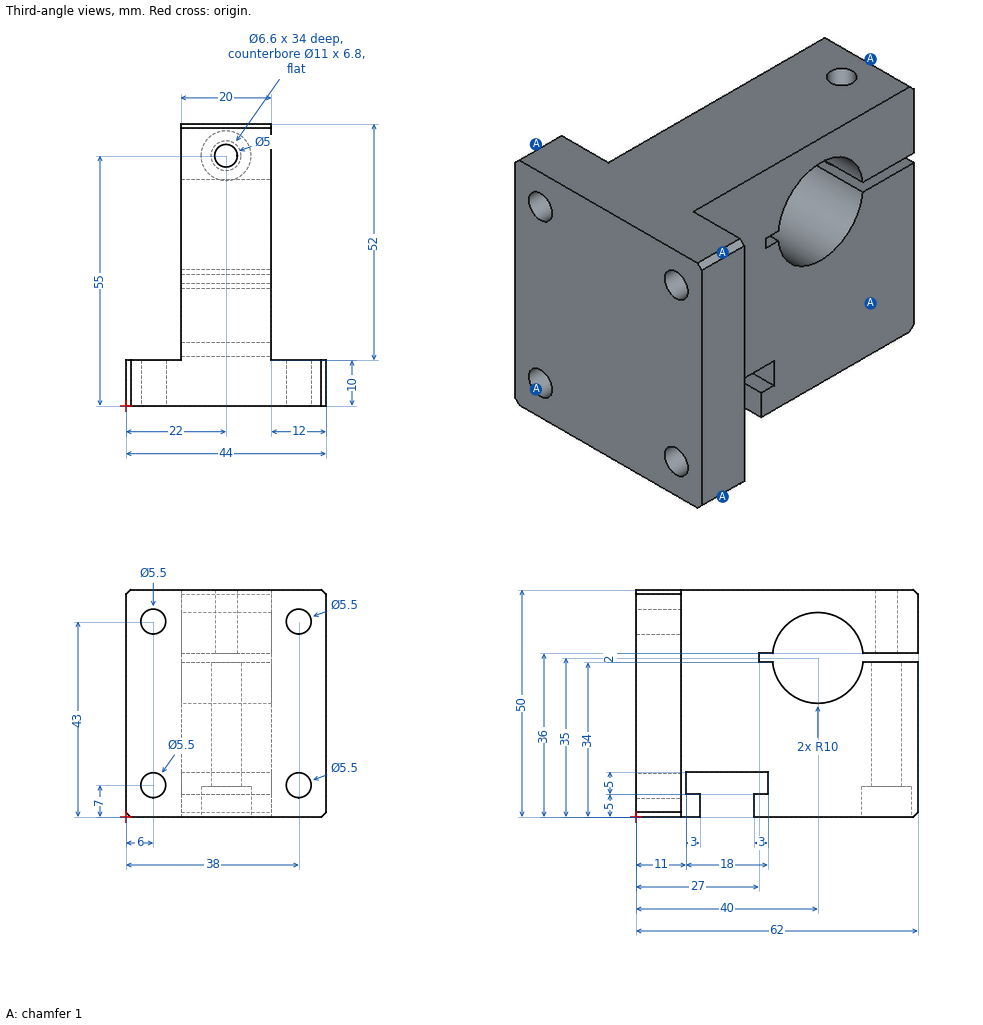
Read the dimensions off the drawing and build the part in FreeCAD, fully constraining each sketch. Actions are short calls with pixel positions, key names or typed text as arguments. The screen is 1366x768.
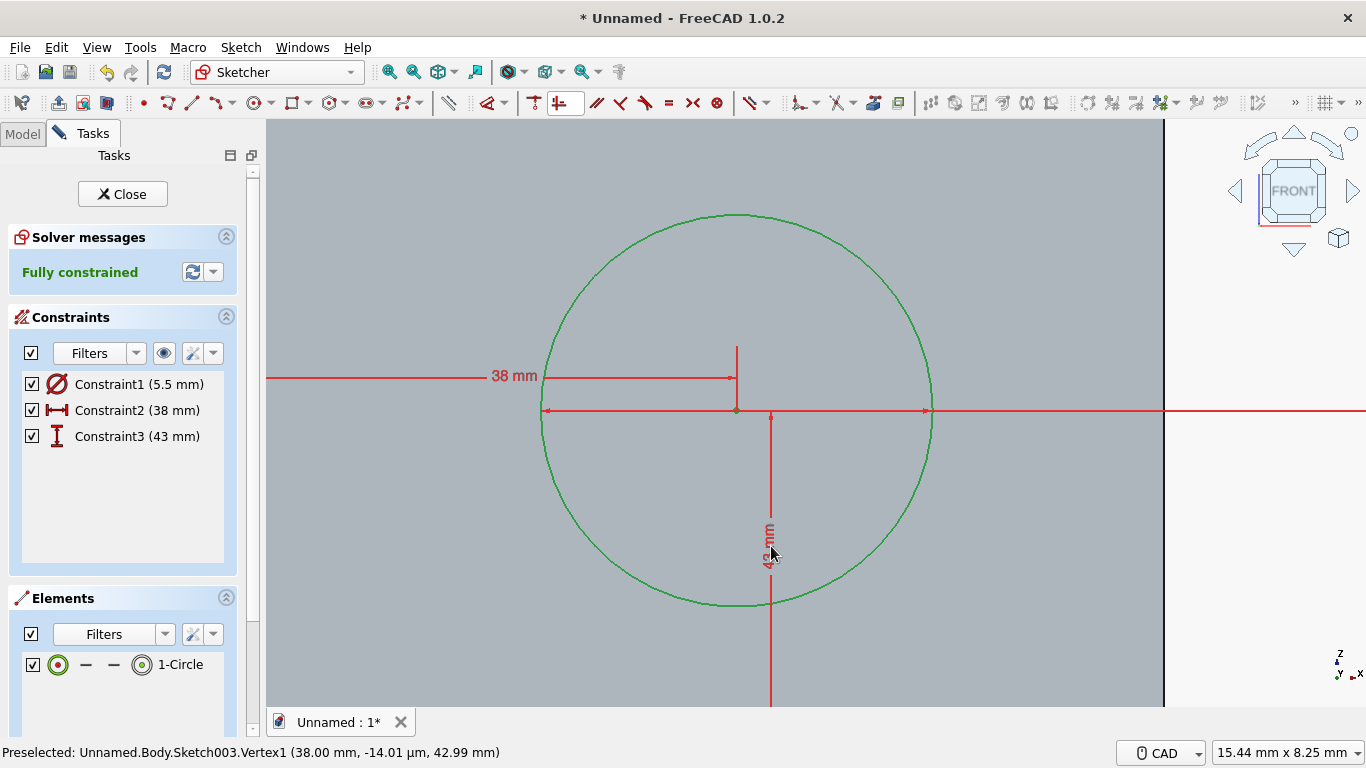
click(123, 194)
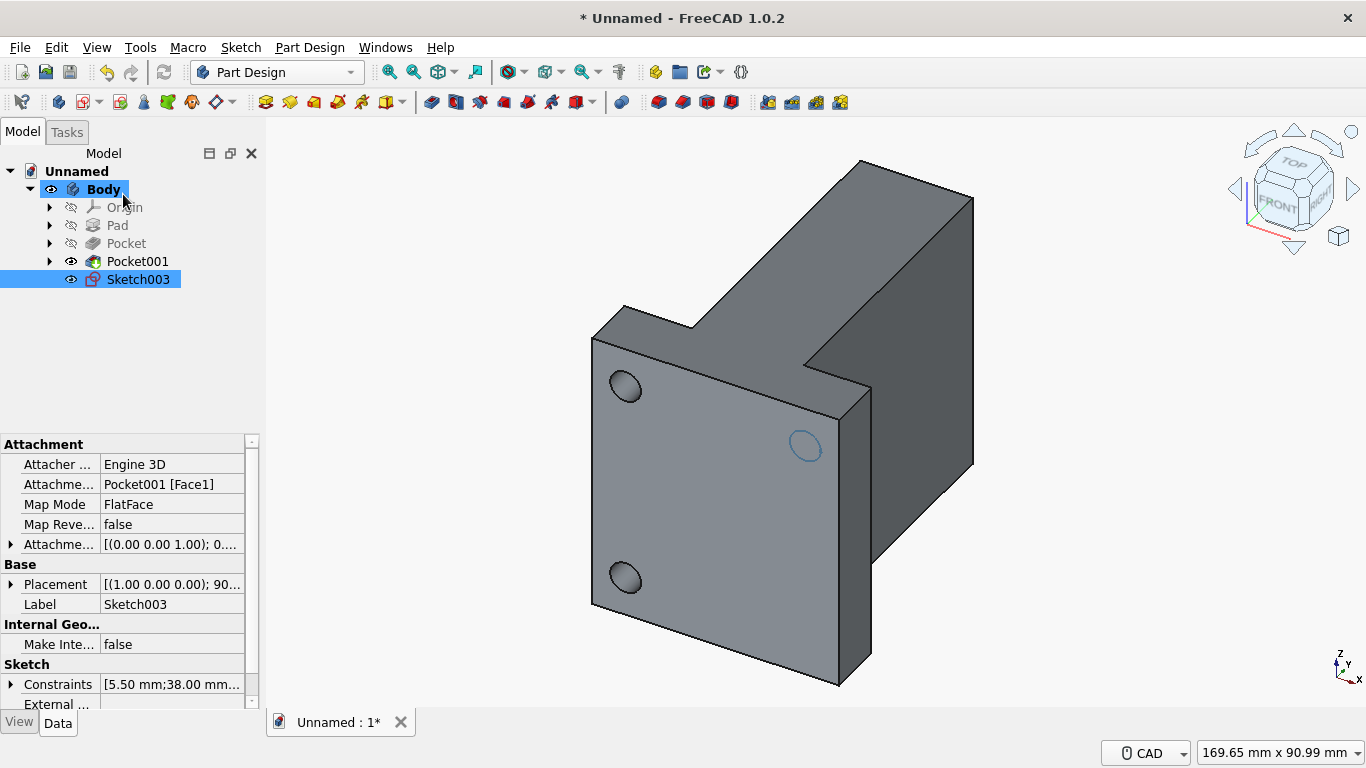
click(432, 102)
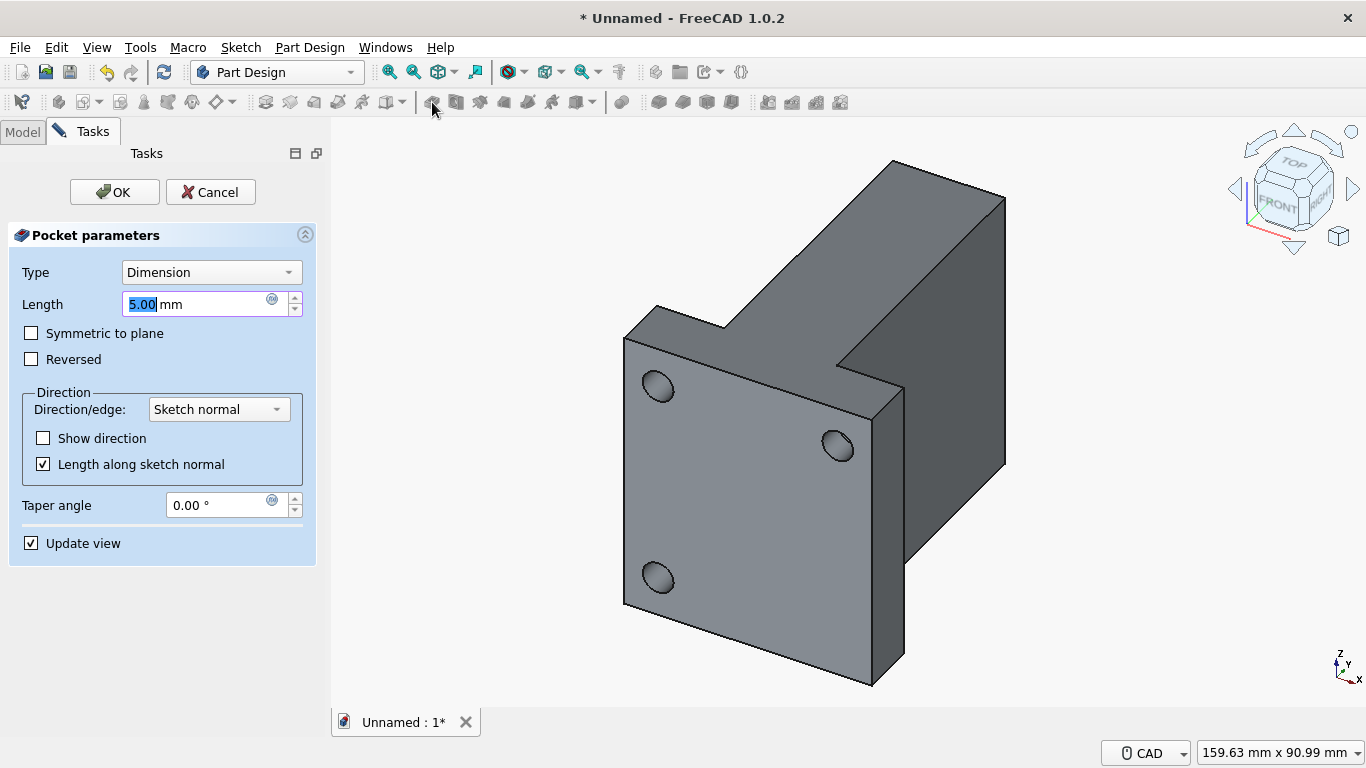
click(212, 272)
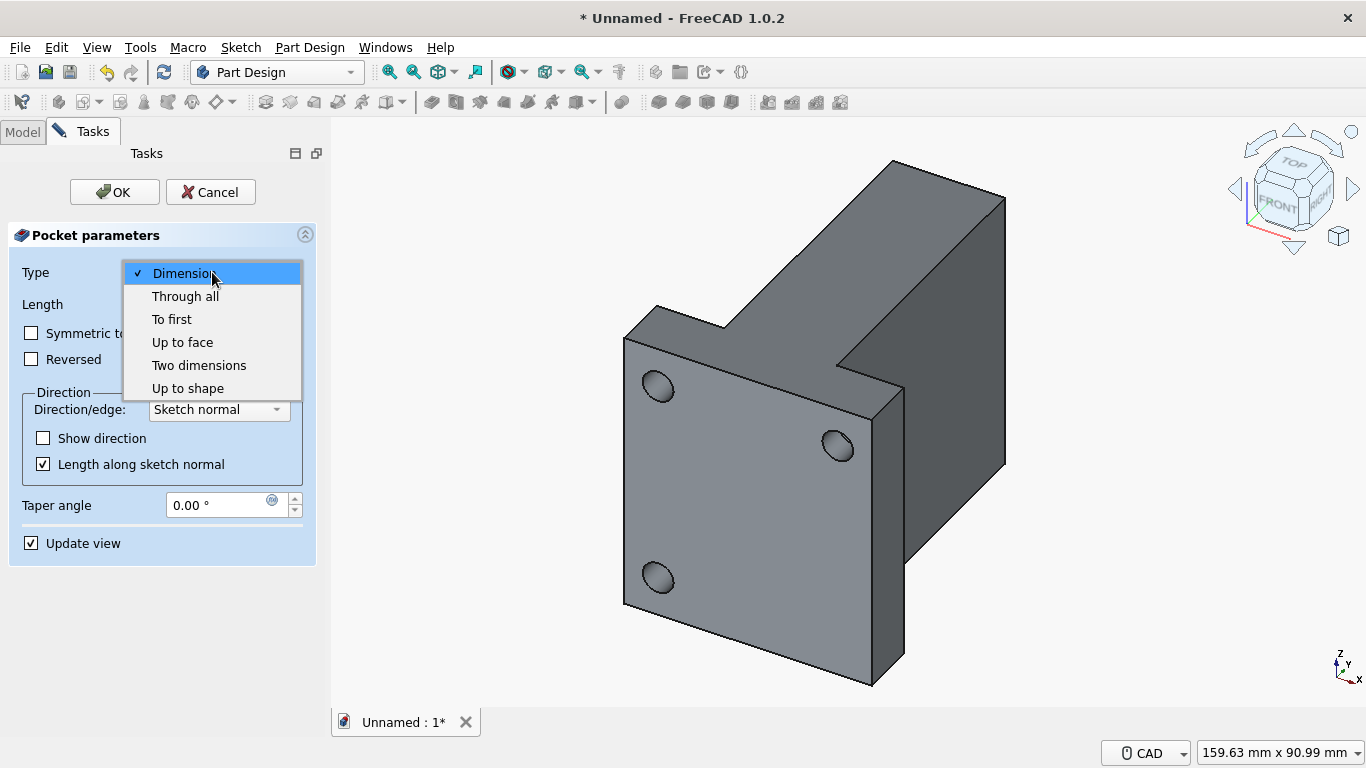
click(212, 320)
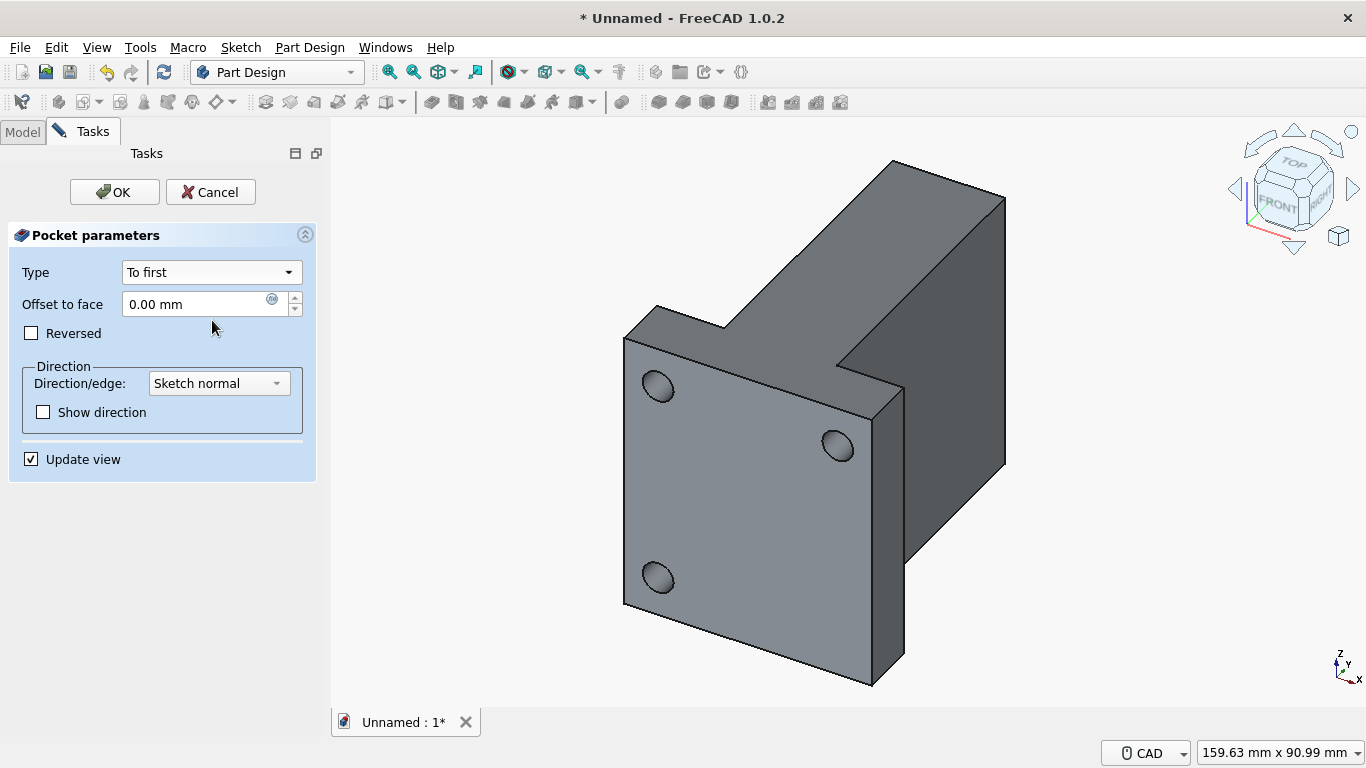
click(115, 192)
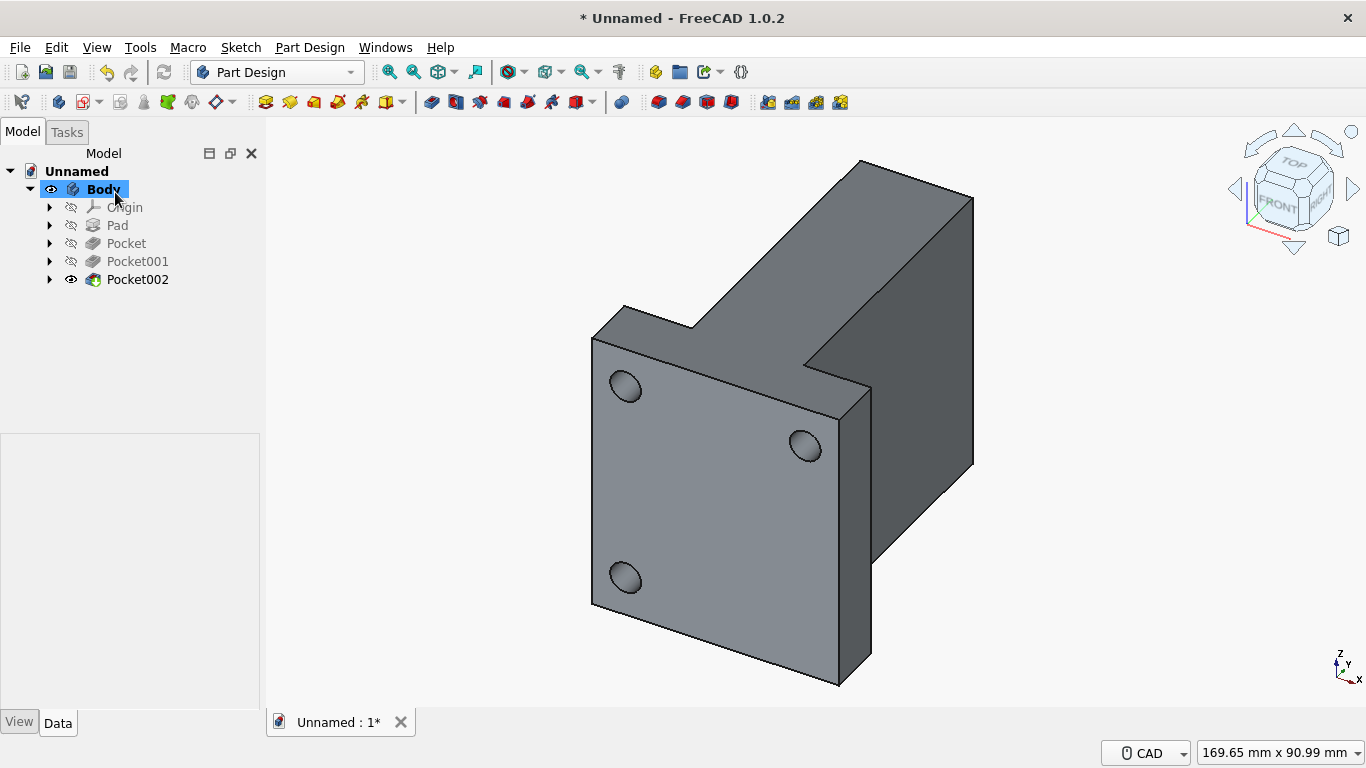
click(84, 102)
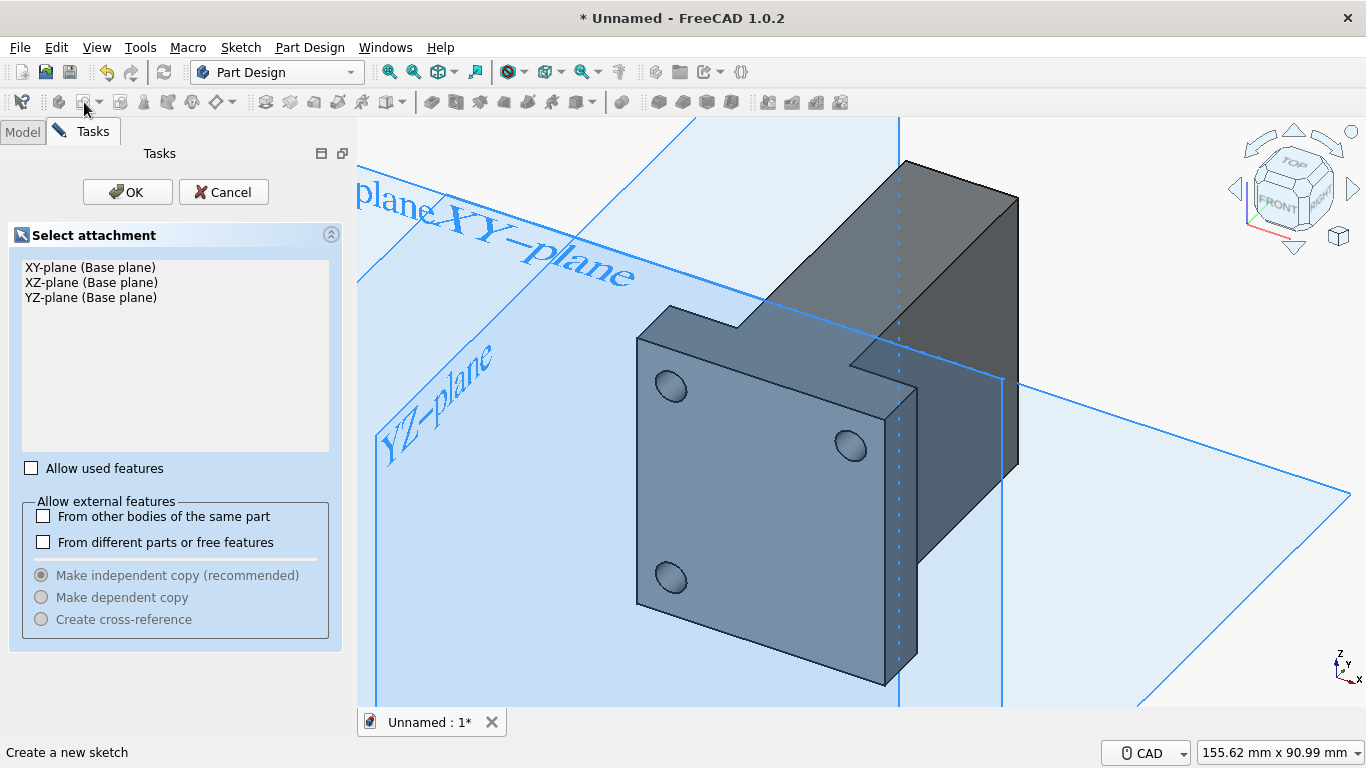
click(82, 282)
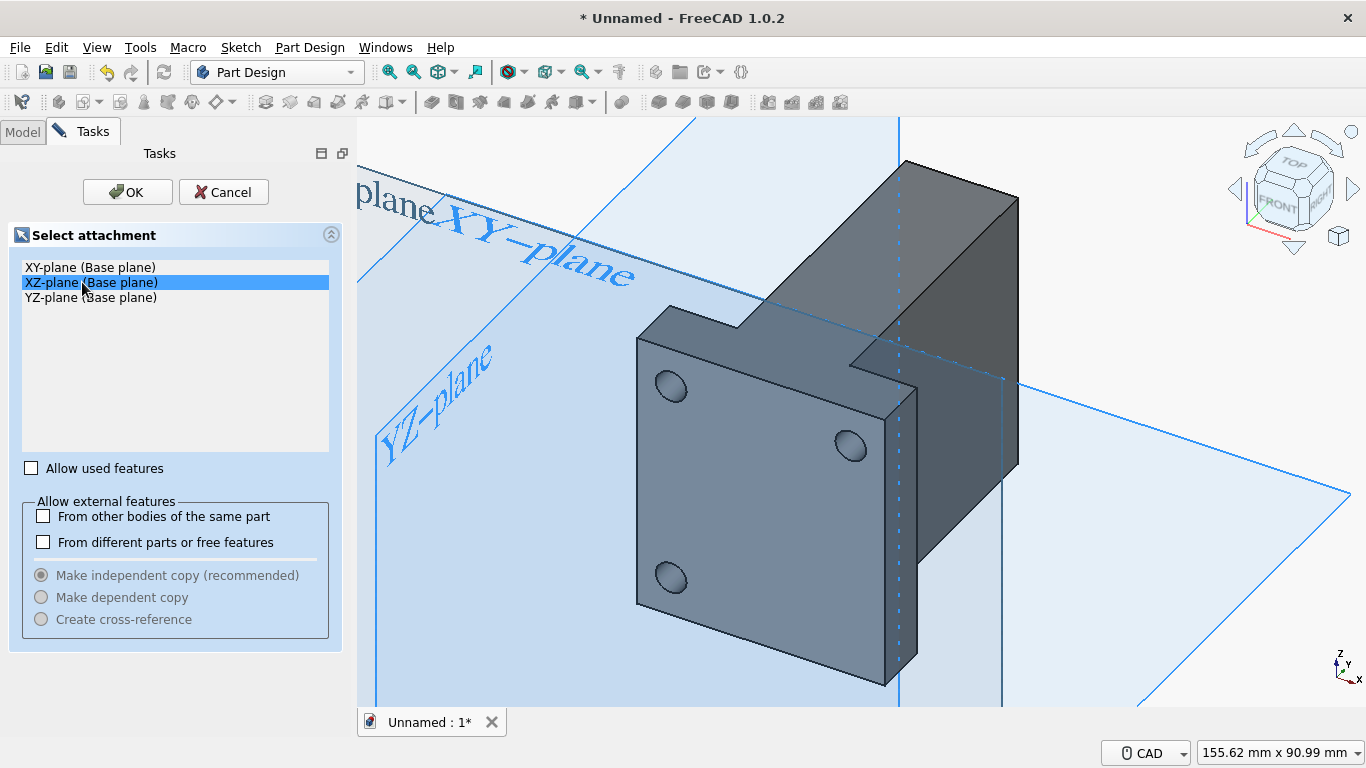
click(128, 192)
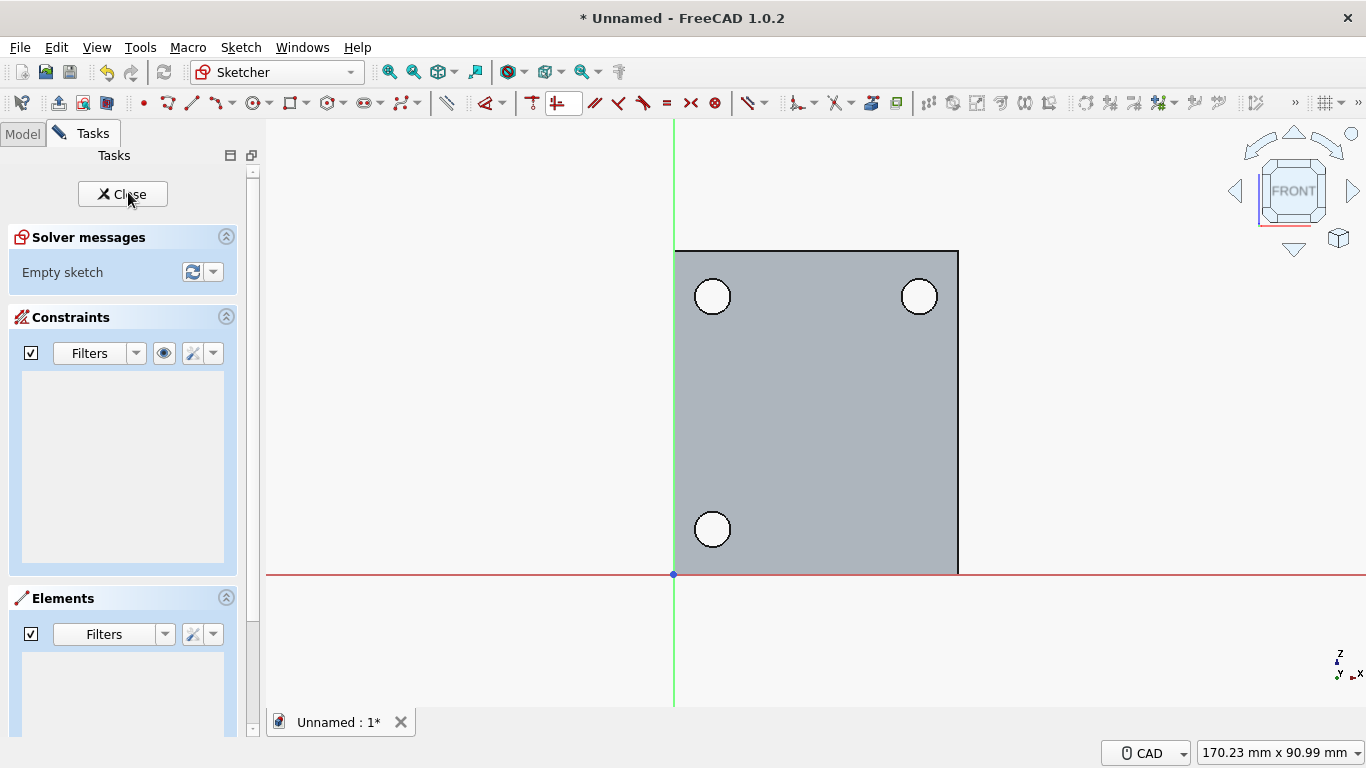
scroll(937, 541, up, 12)